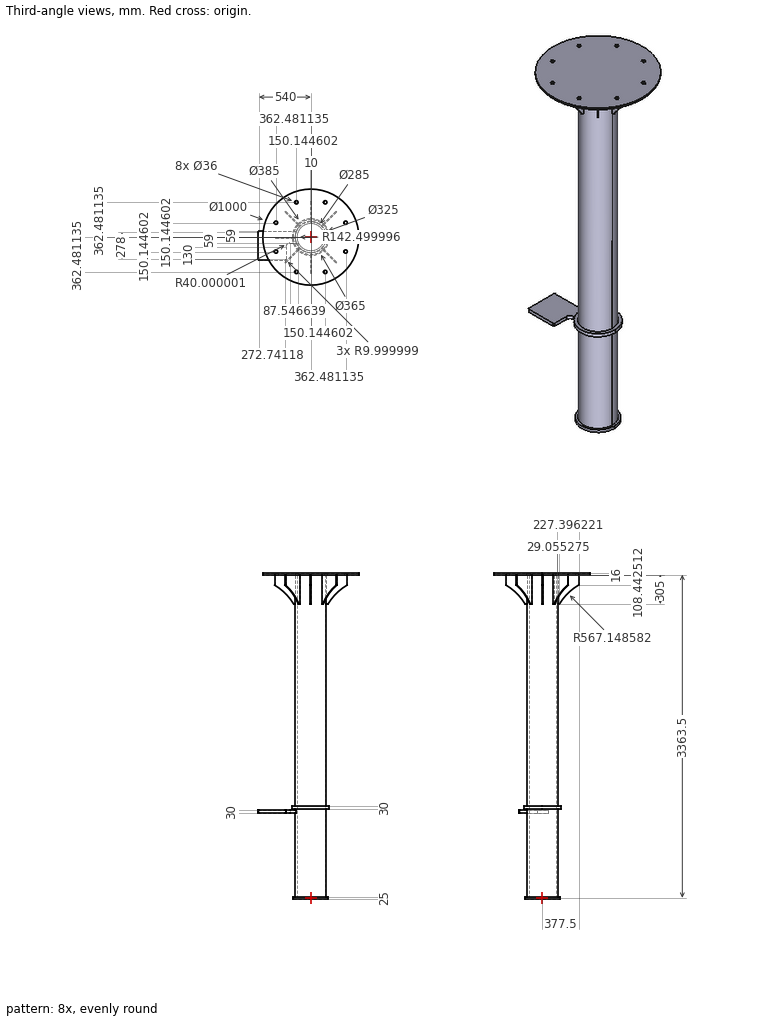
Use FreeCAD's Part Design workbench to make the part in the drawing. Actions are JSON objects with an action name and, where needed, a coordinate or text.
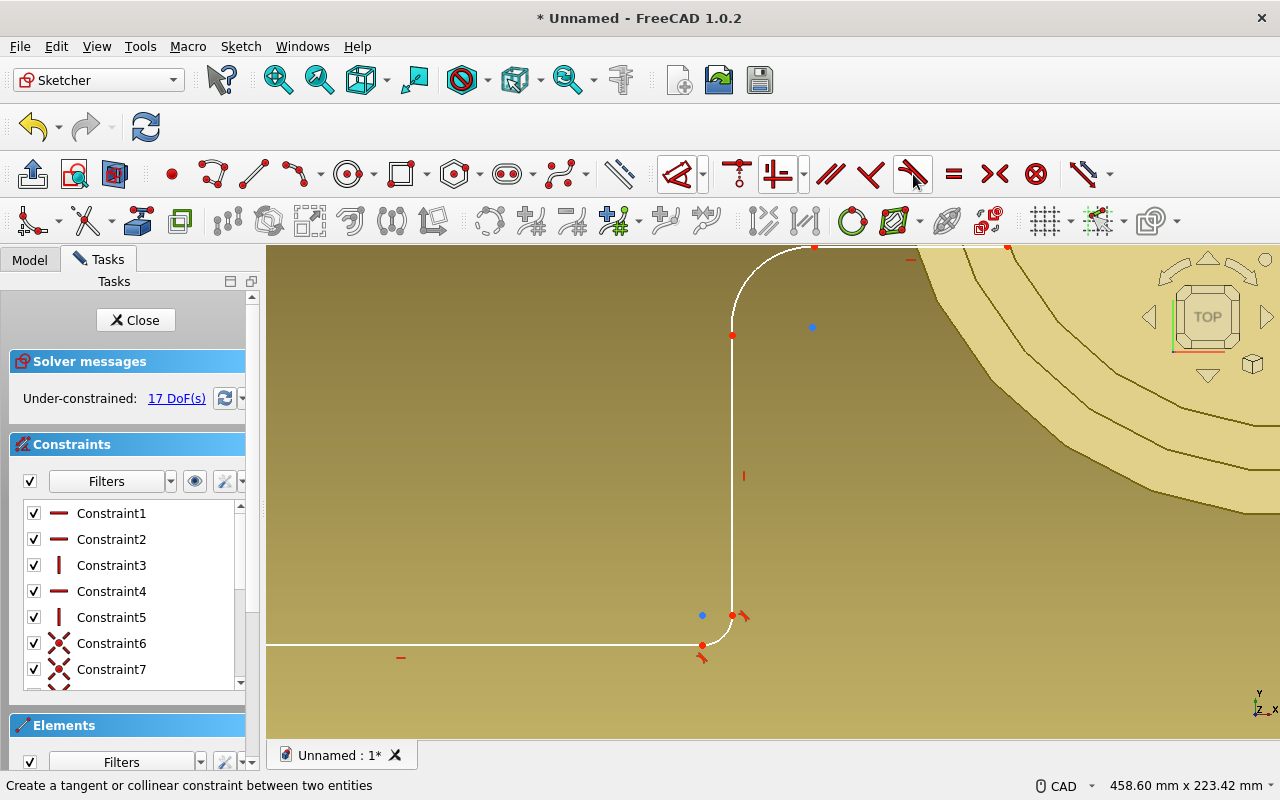
{"action": "left_click", "coordinate": [522, 645]}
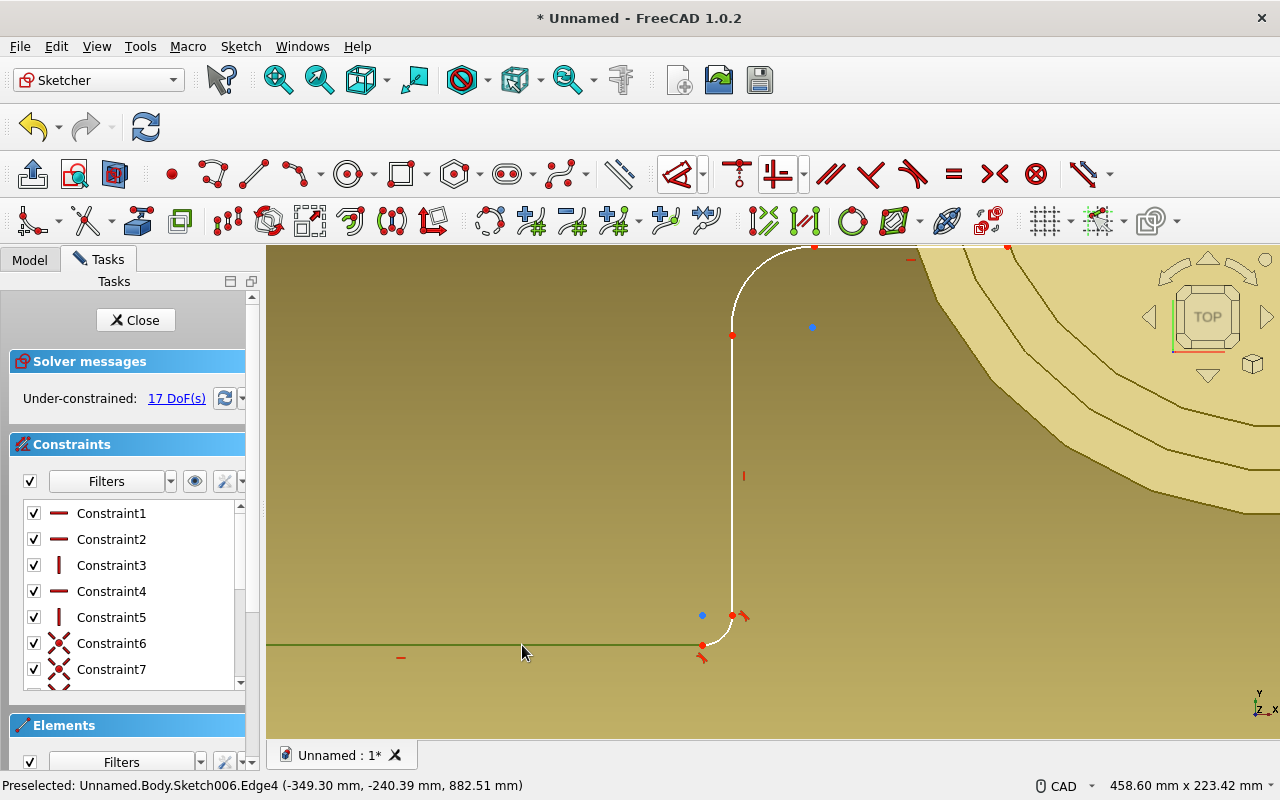
{"action": "scroll", "coordinate": [719, 638], "scroll_direction": "down", "scroll_amount": 4}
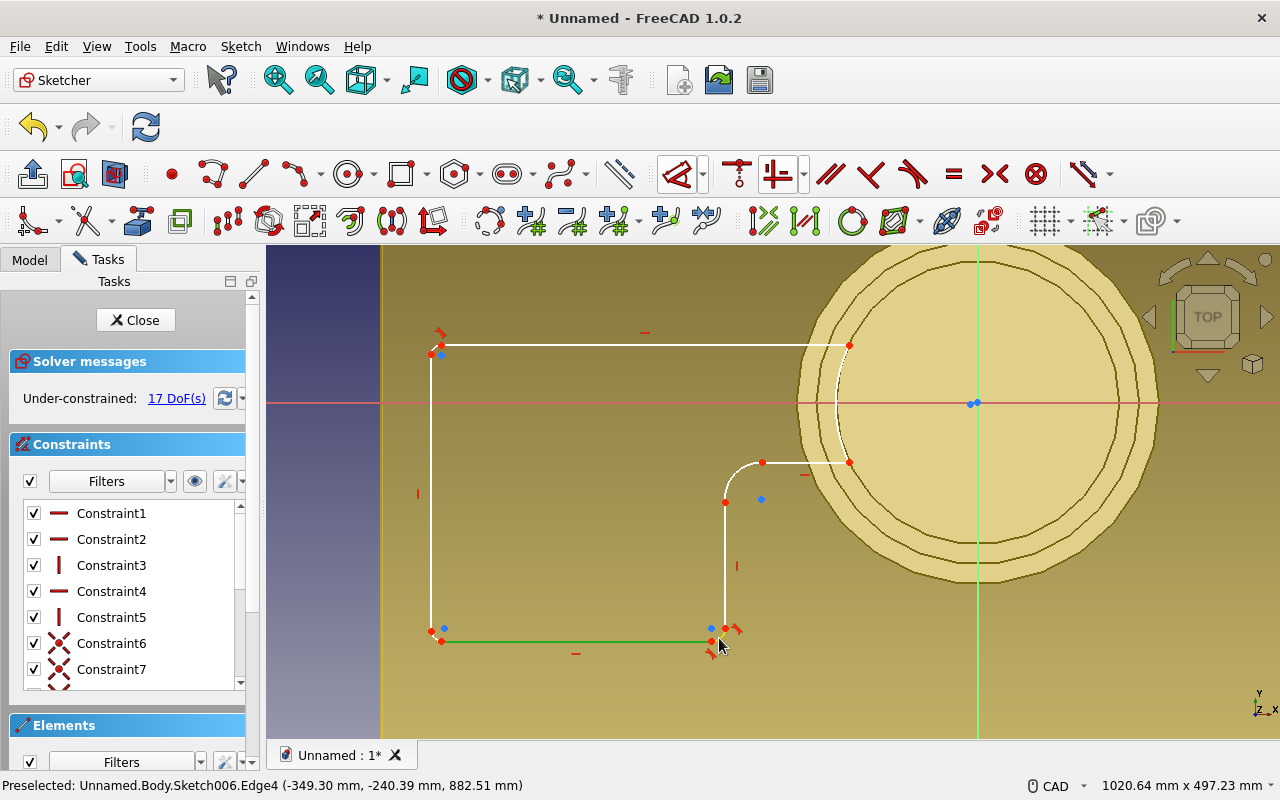
{"action": "scroll", "coordinate": [433, 636], "scroll_direction": "up", "scroll_amount": 6}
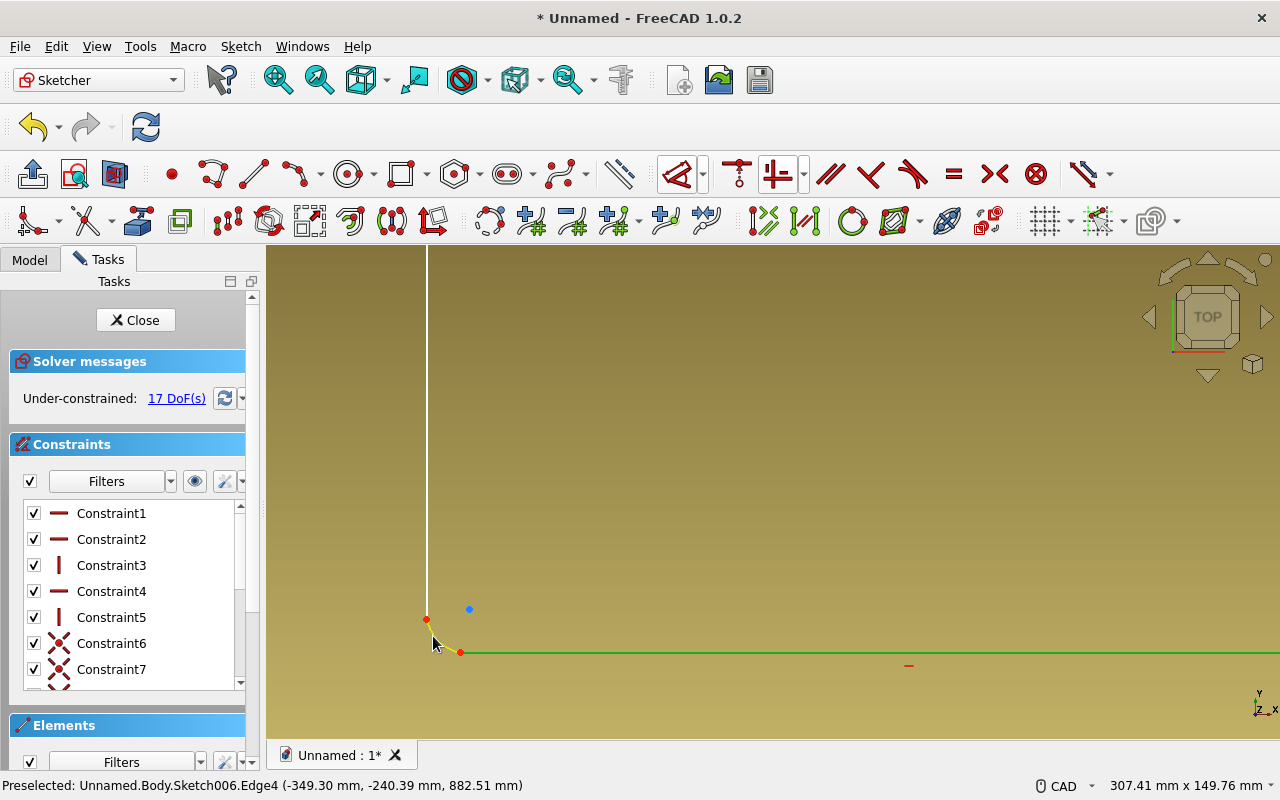
{"action": "left_click", "coordinate": [433, 633]}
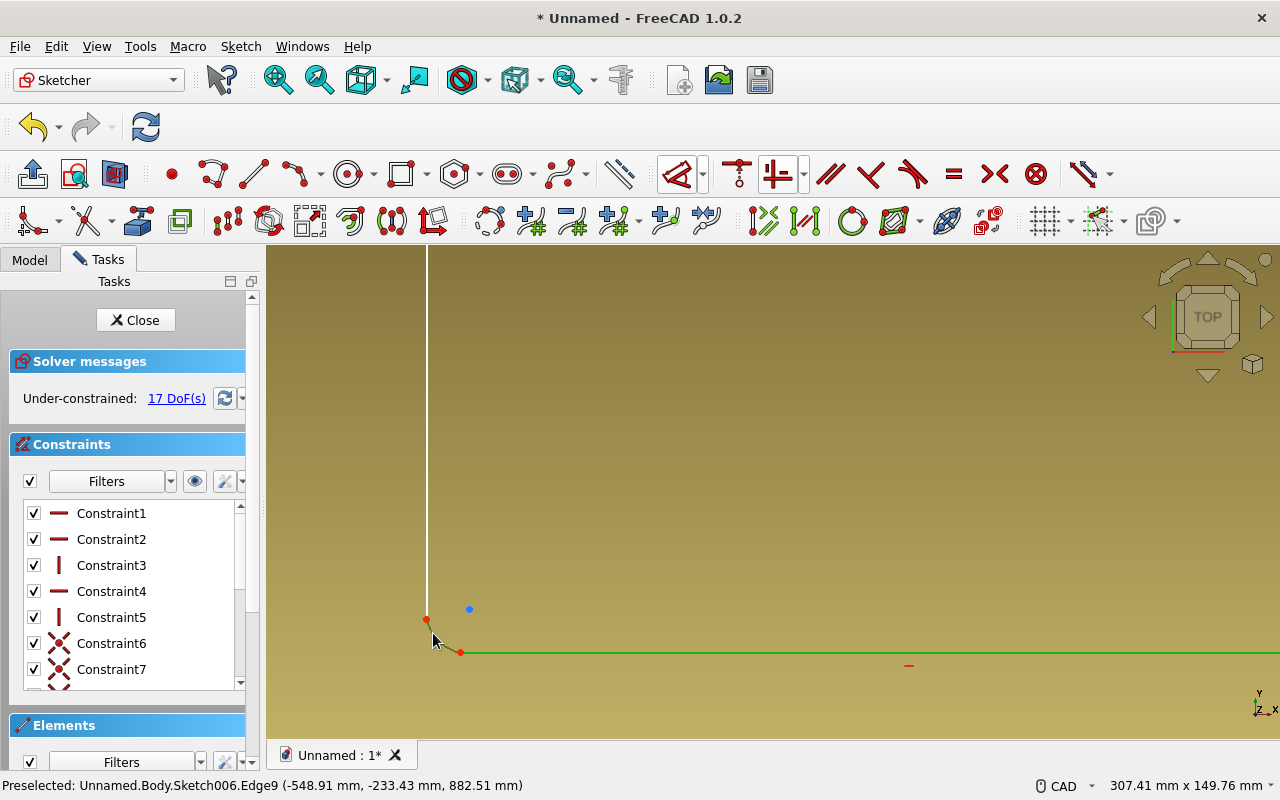
{"action": "left_click", "coordinate": [913, 174]}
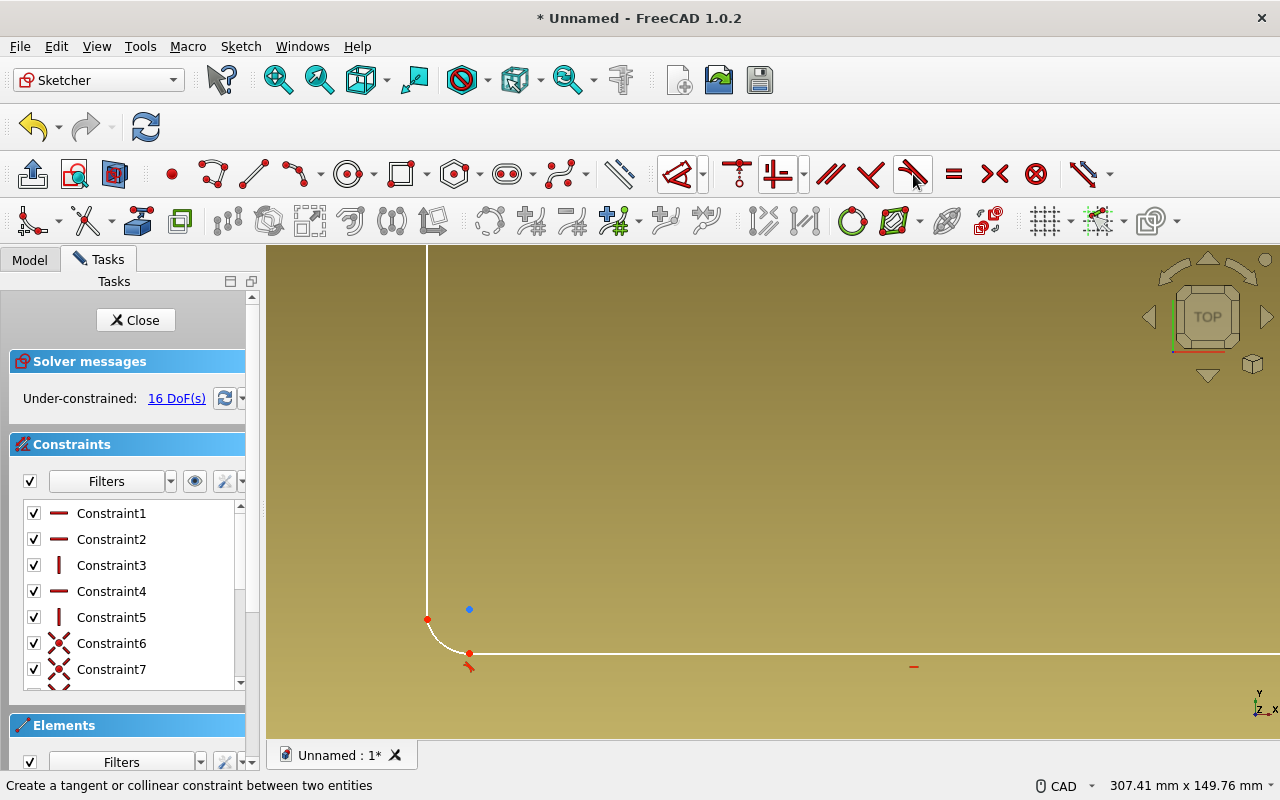
{"action": "left_click", "coordinate": [427, 344]}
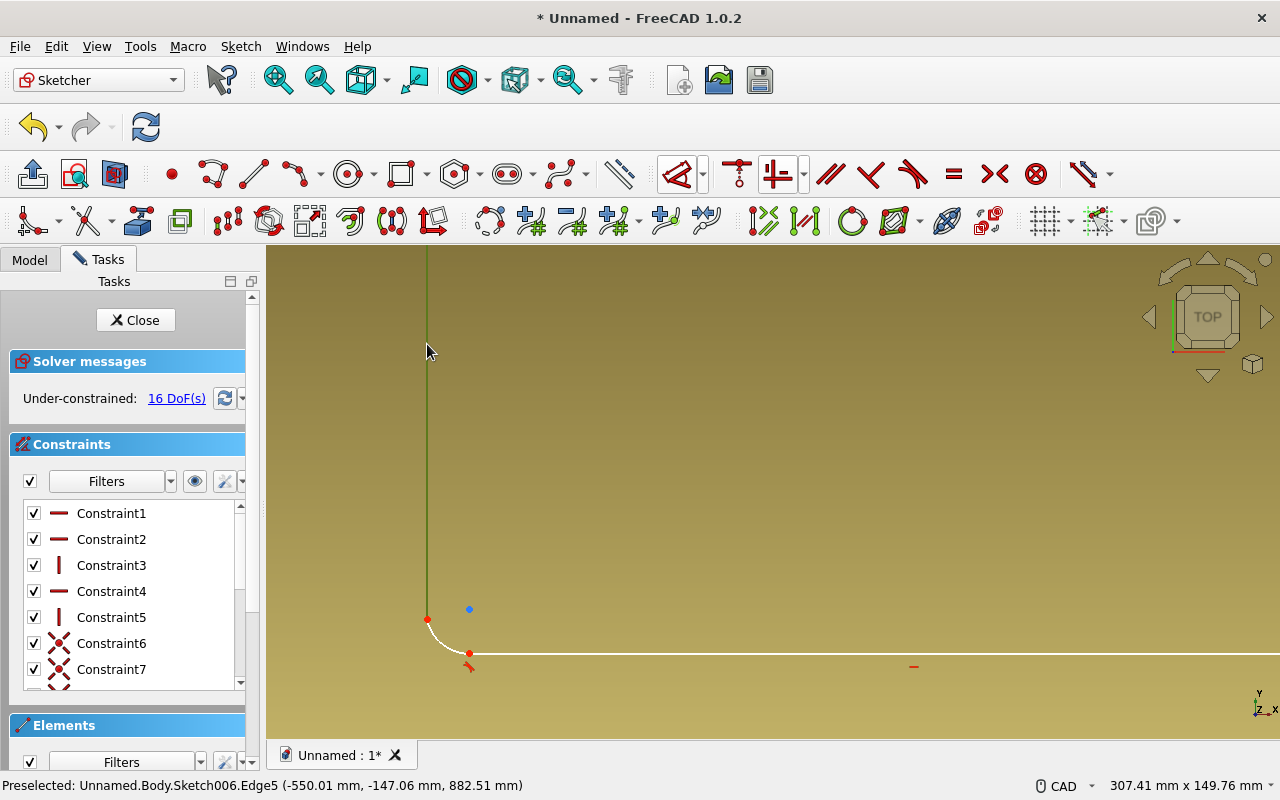
{"action": "left_click", "coordinate": [434, 636]}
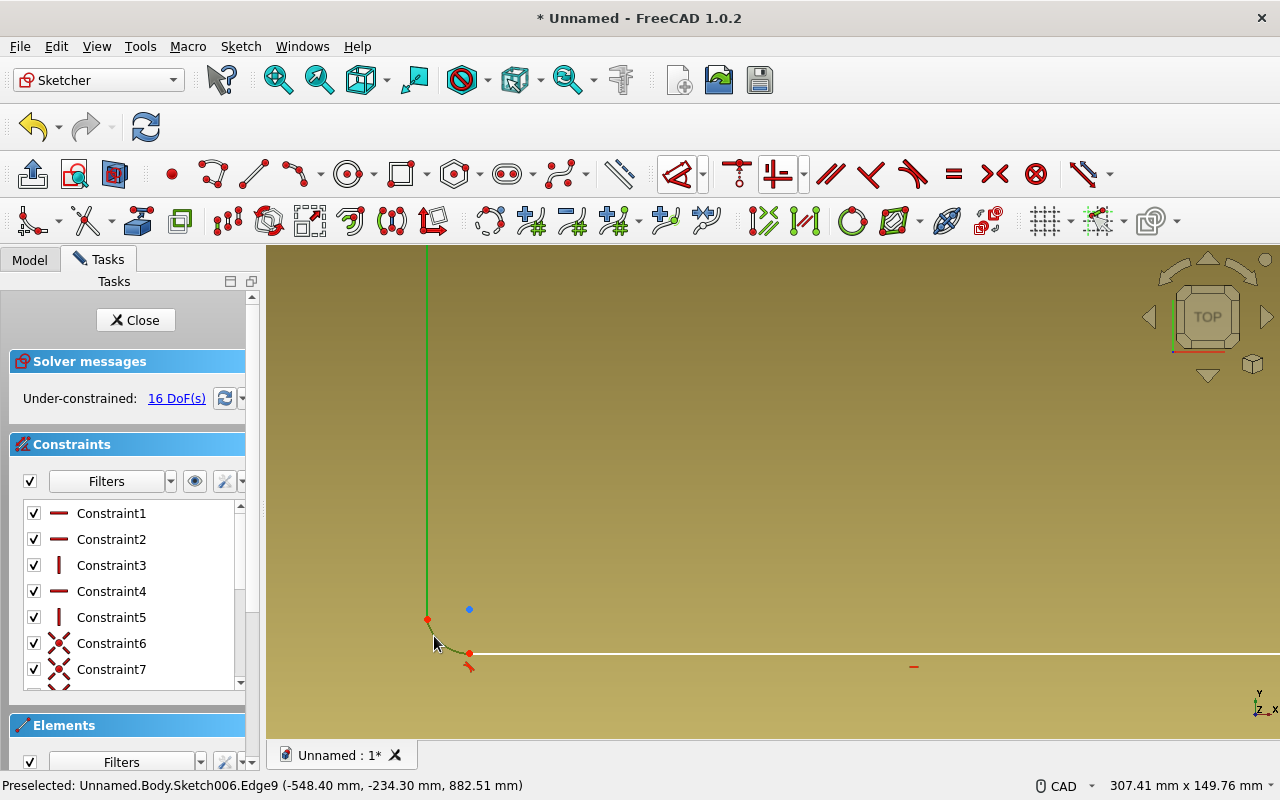
{"action": "left_click", "coordinate": [913, 174]}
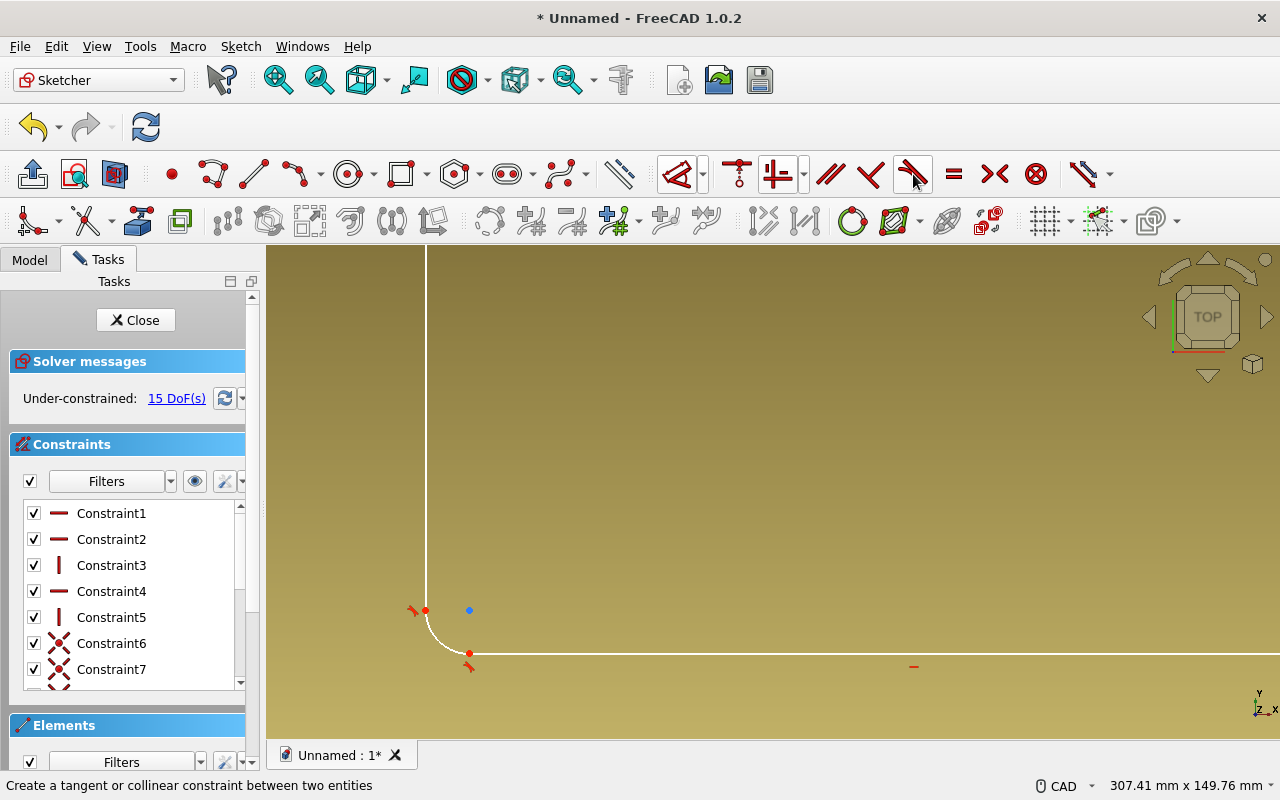
{"action": "left_click", "coordinate": [426, 337]}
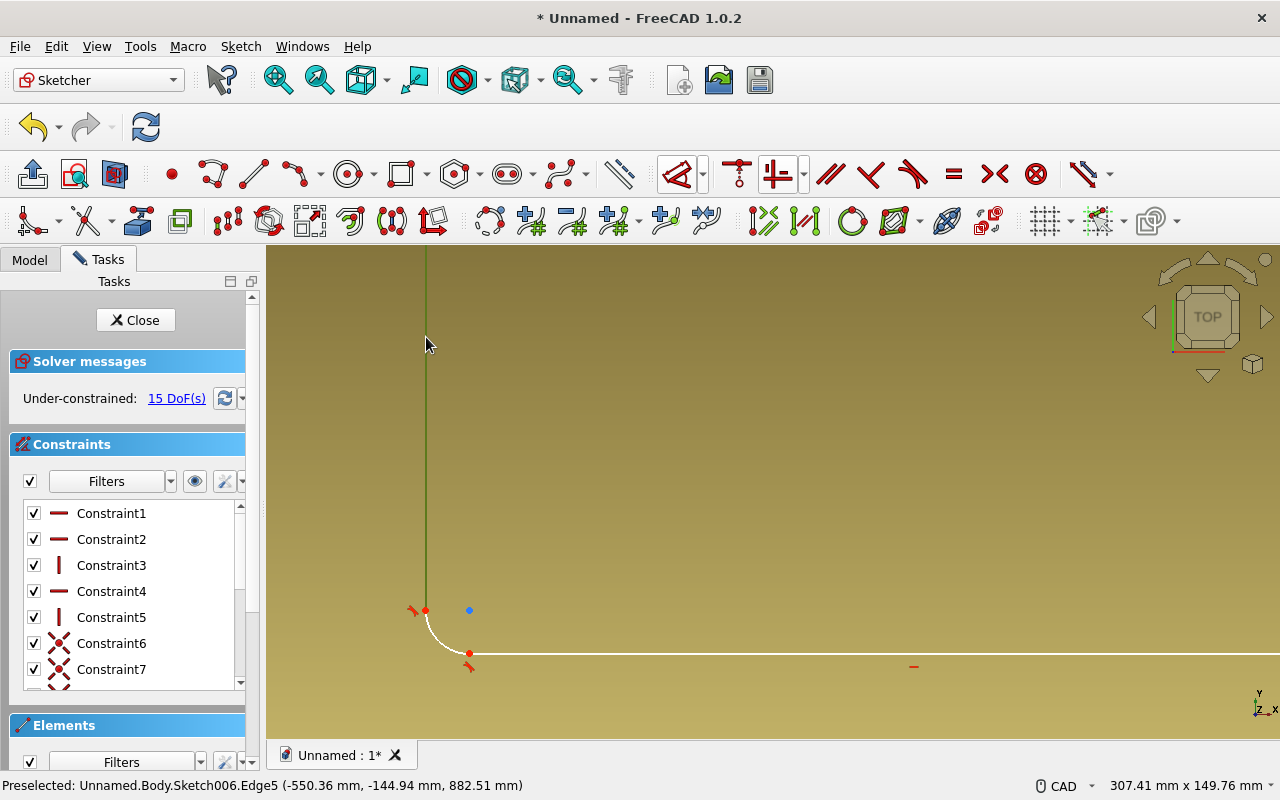
{"action": "scroll", "coordinate": [433, 636], "scroll_direction": "down", "scroll_amount": 6}